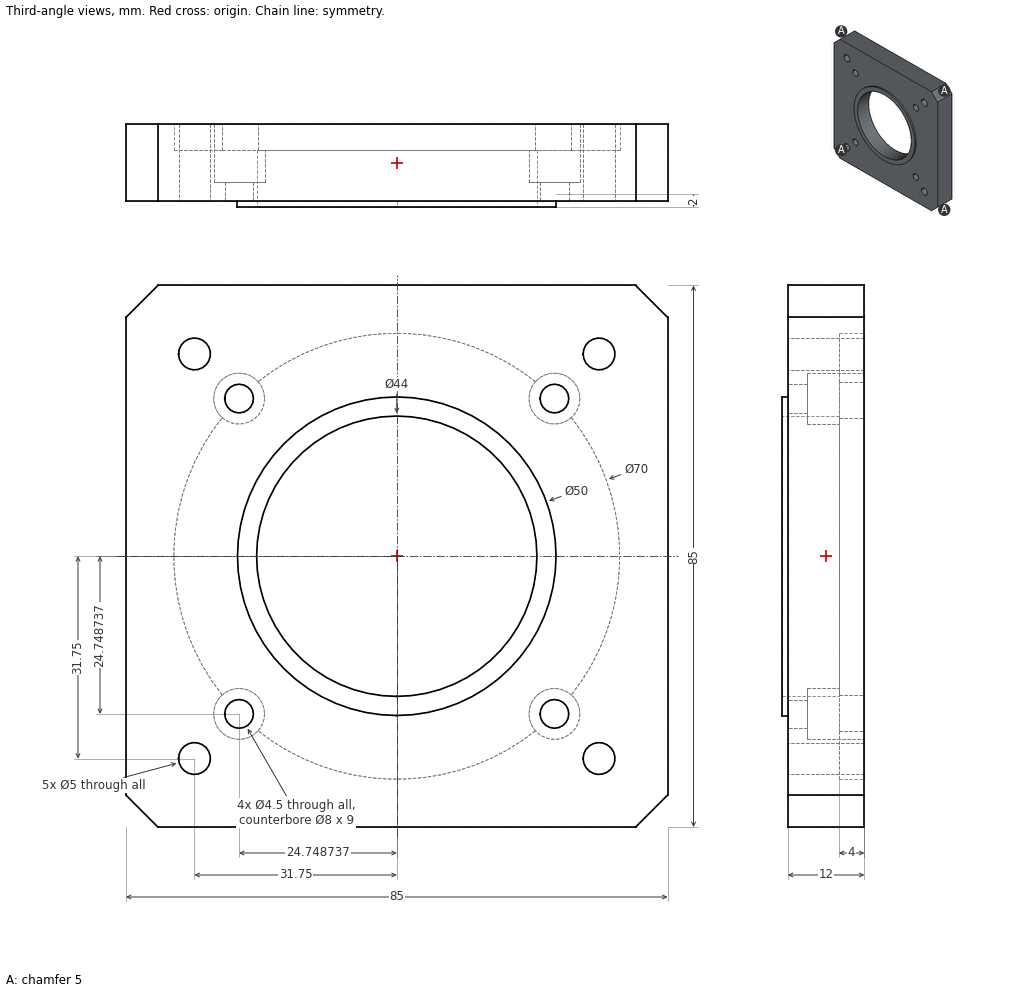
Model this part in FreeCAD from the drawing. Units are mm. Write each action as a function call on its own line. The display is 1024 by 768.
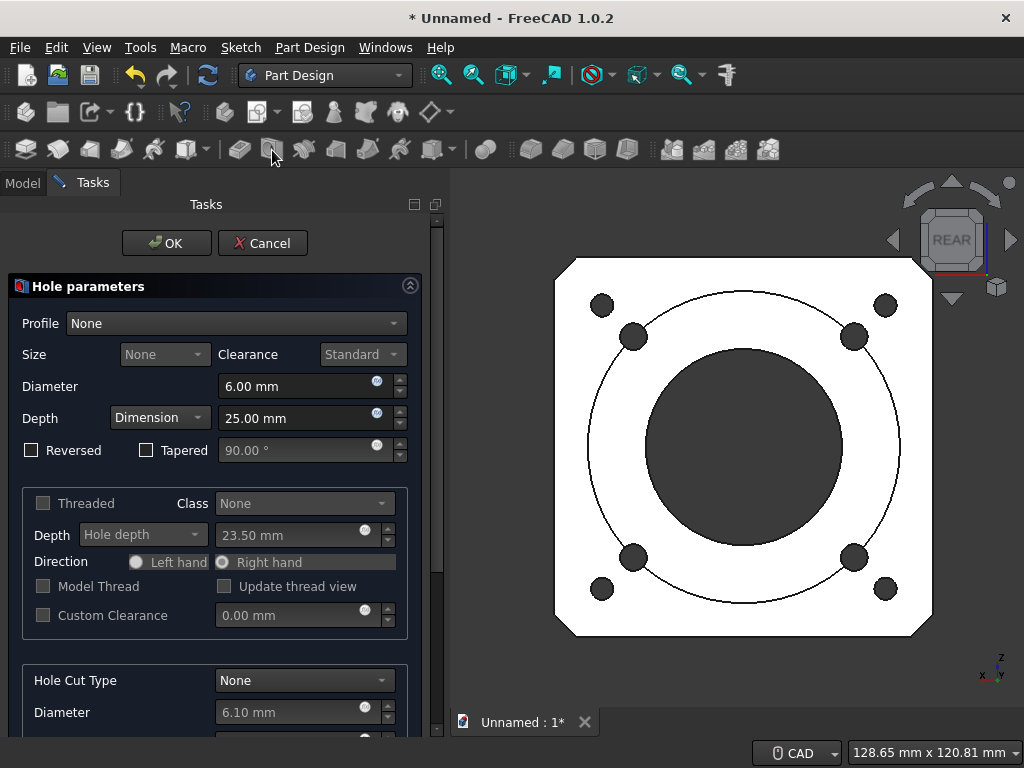
triple_click(305, 386)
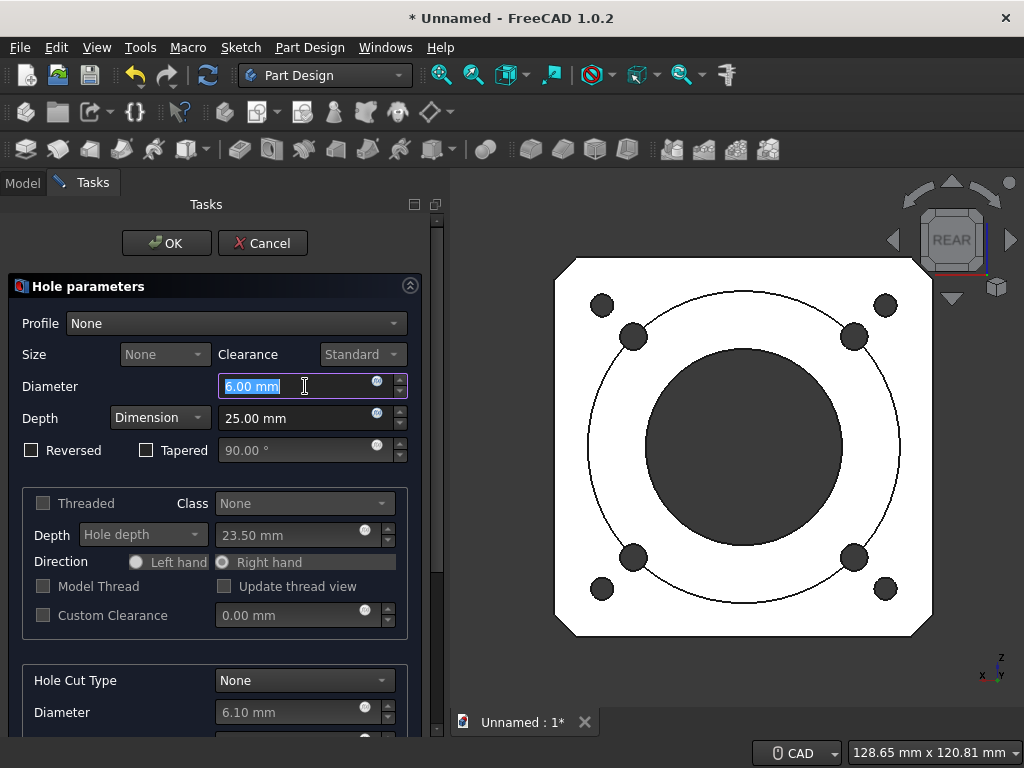
text(4.5)
key(Tab)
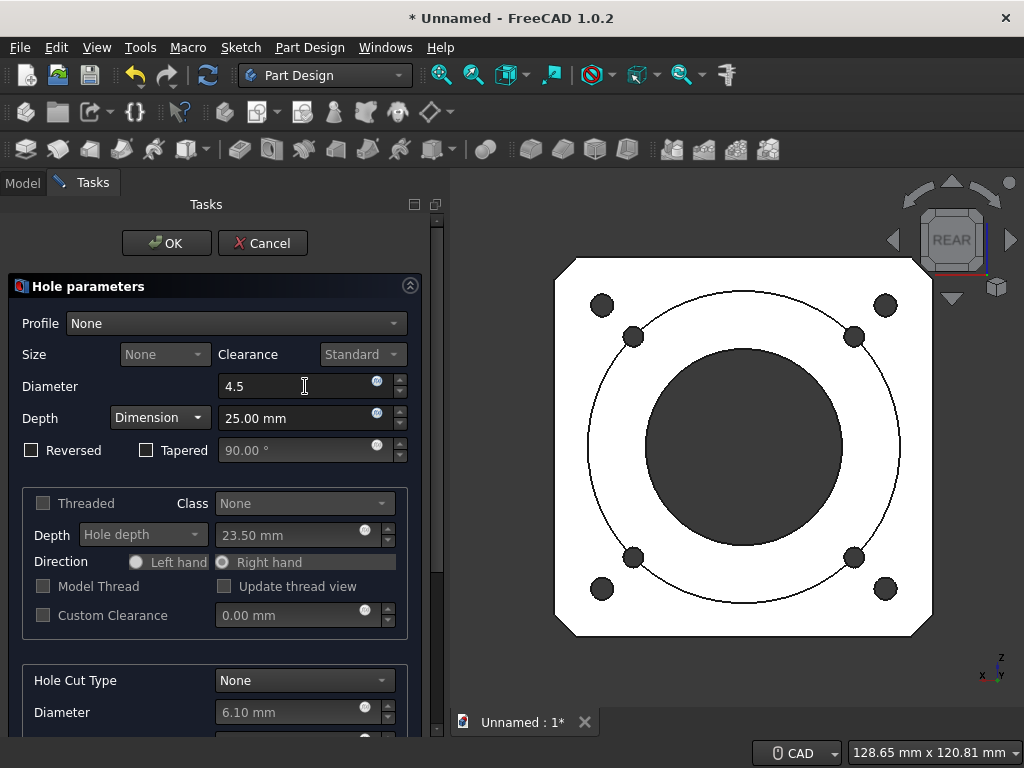
click(161, 418)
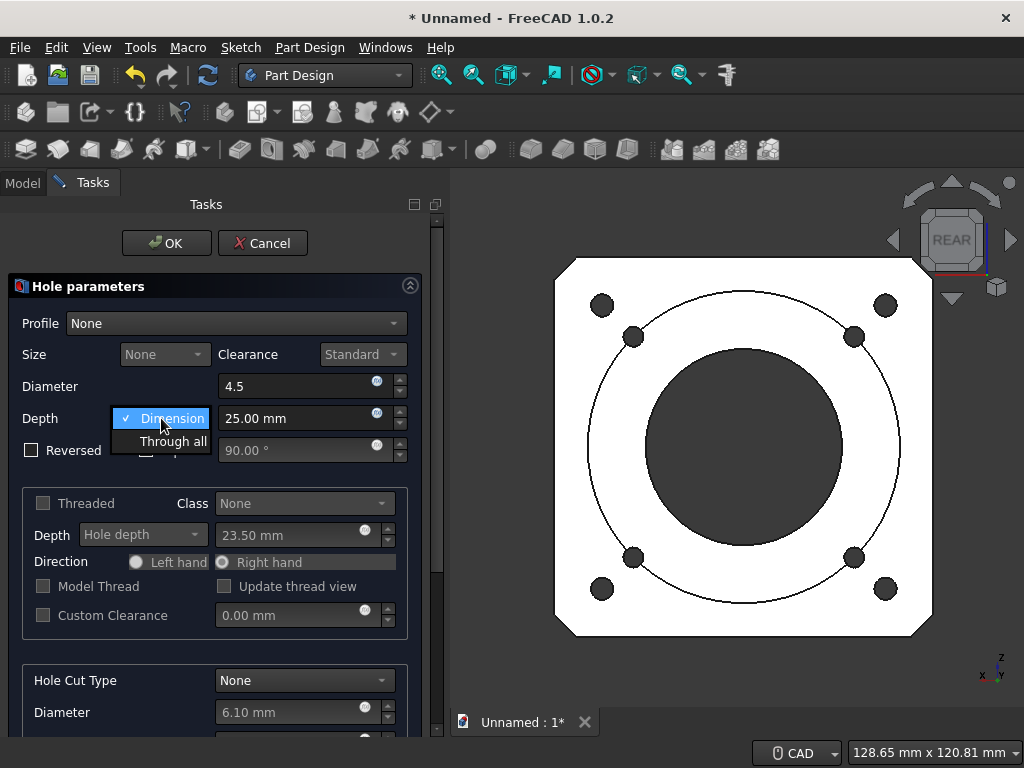
click(160, 442)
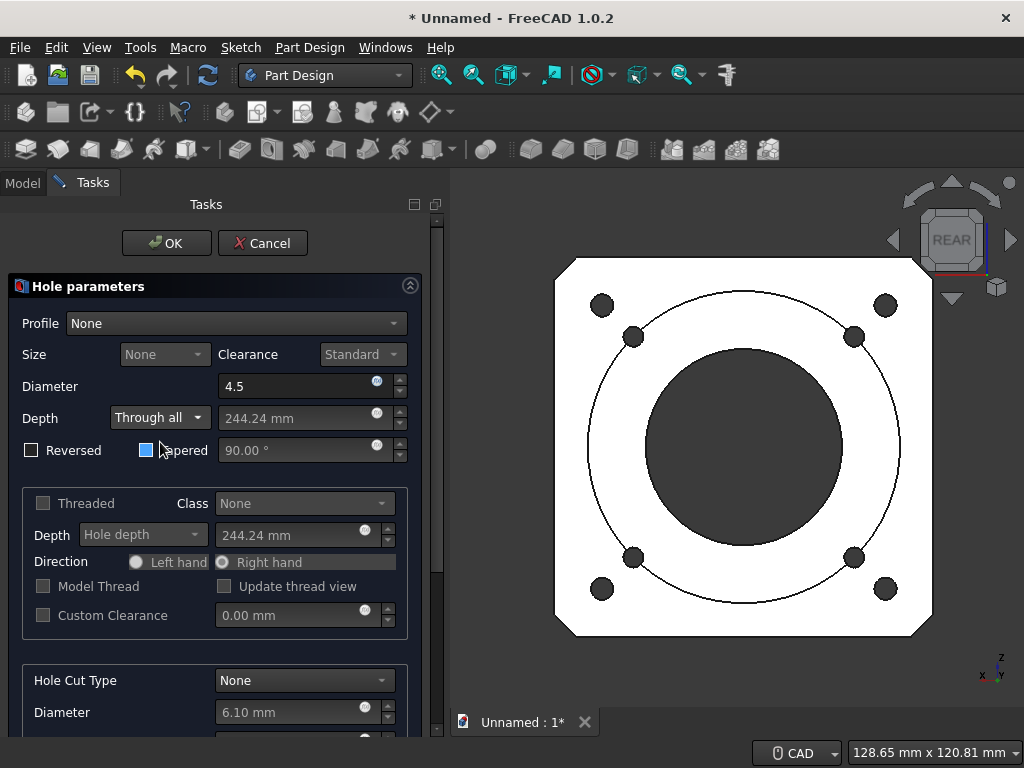
click(306, 680)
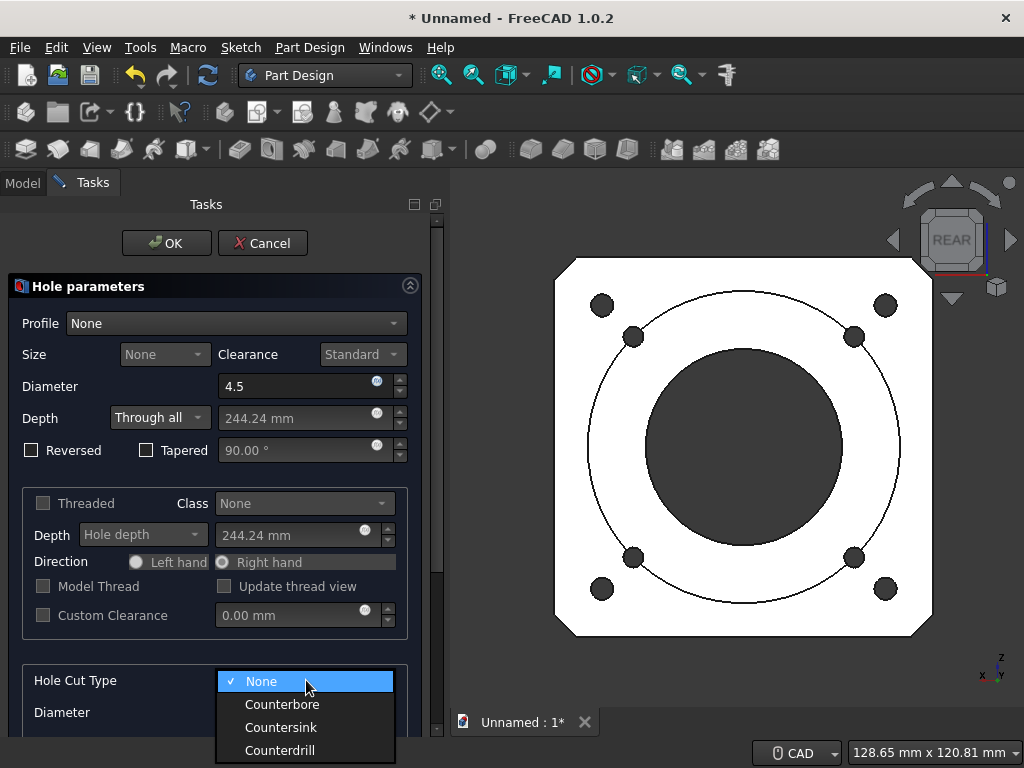
click(304, 704)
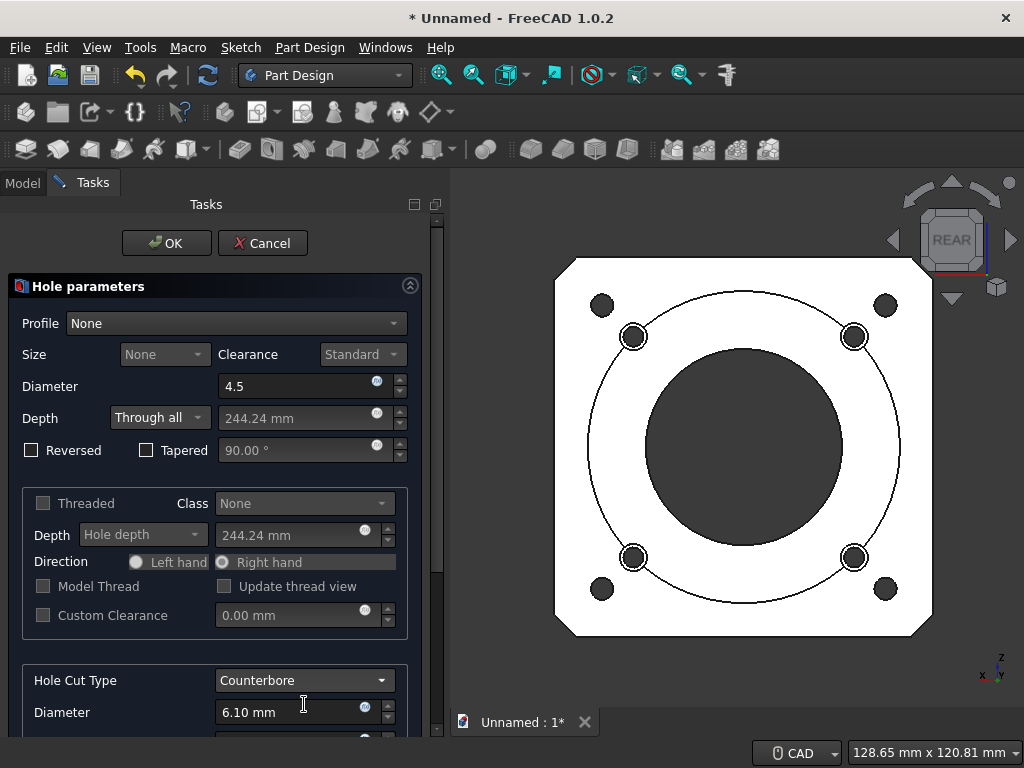
triple_click(298, 712)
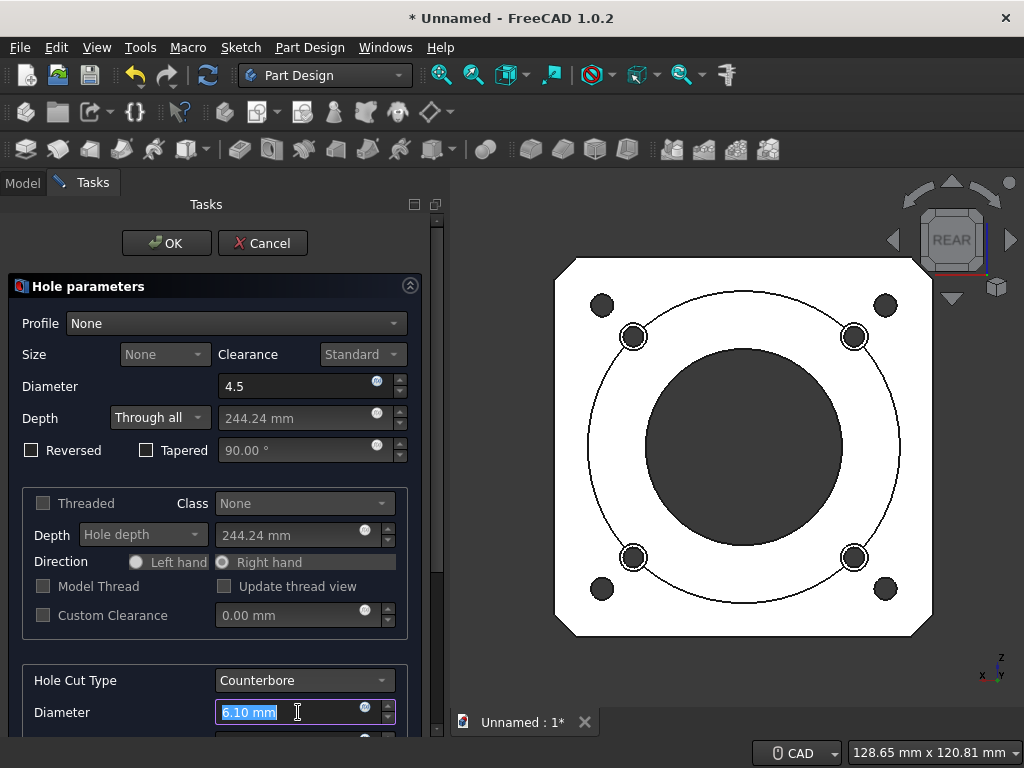
text(8)
key(Tab)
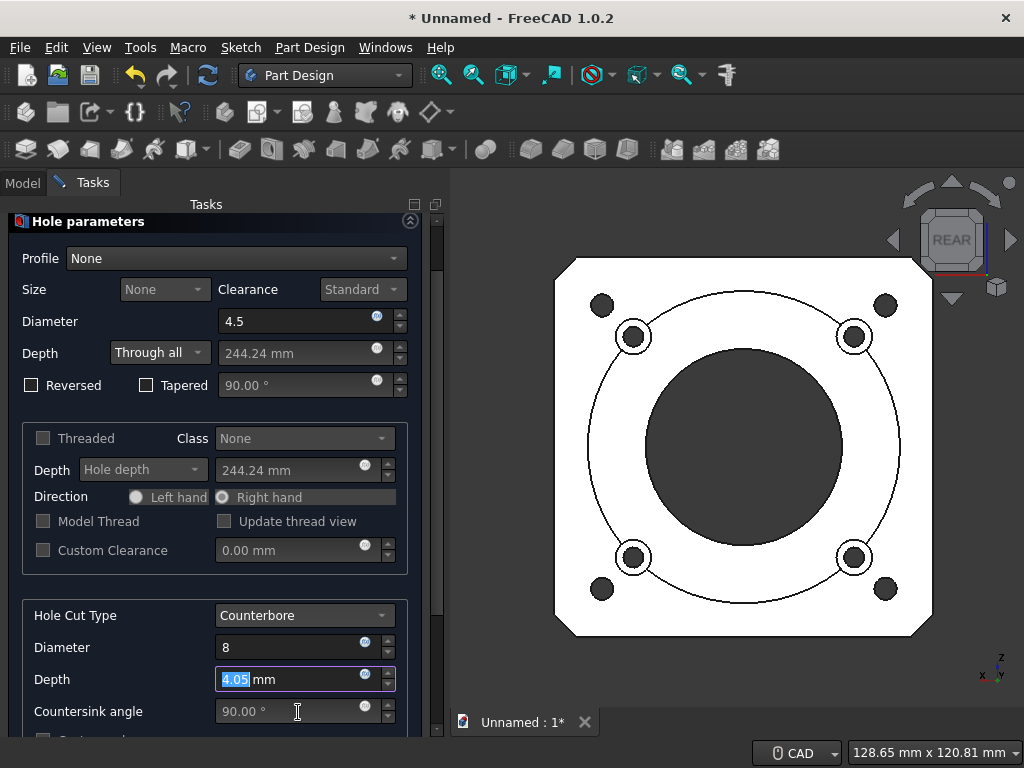
text(9)
key(Tab)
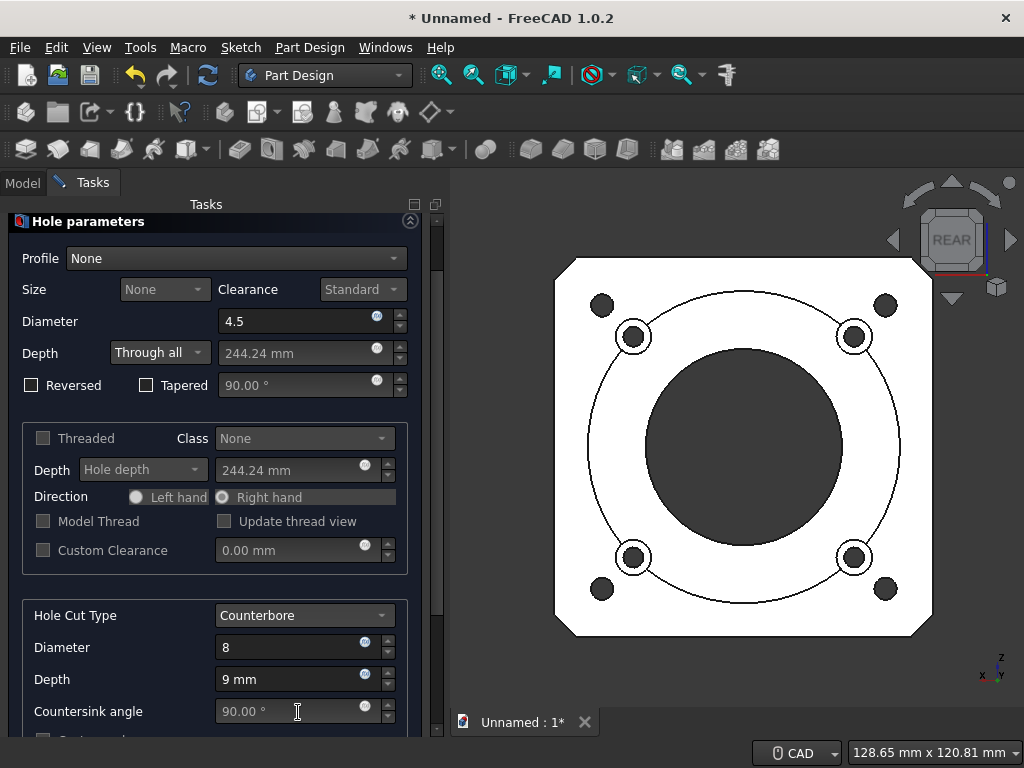
scroll(437, 475, up, 2)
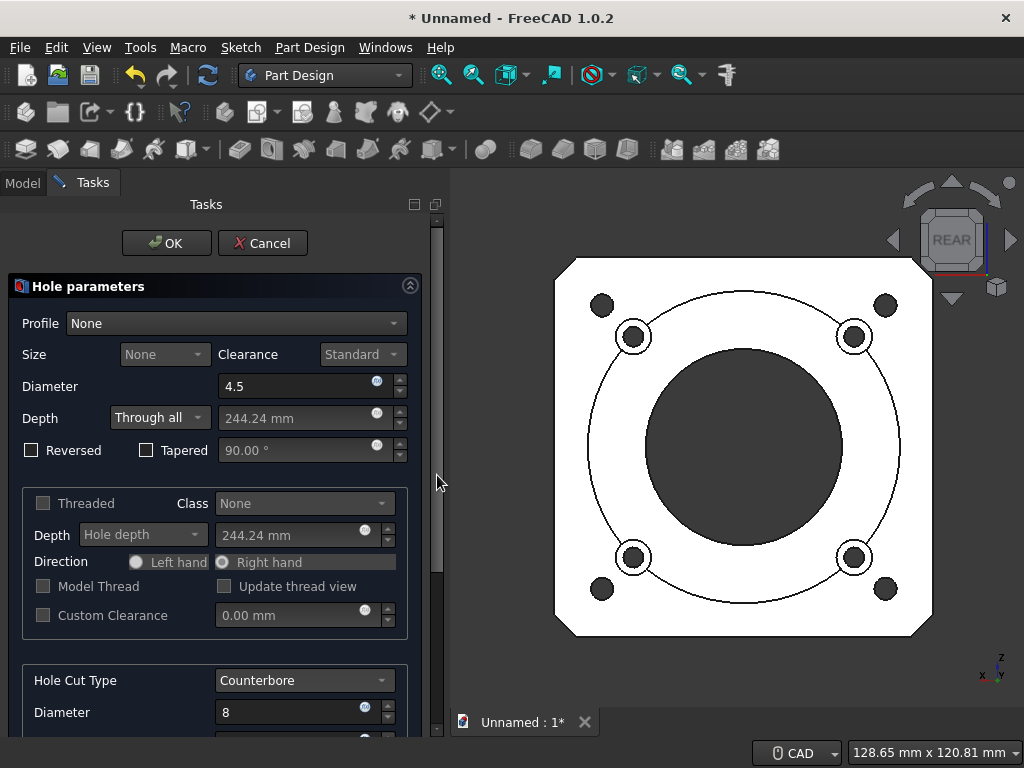
click(167, 243)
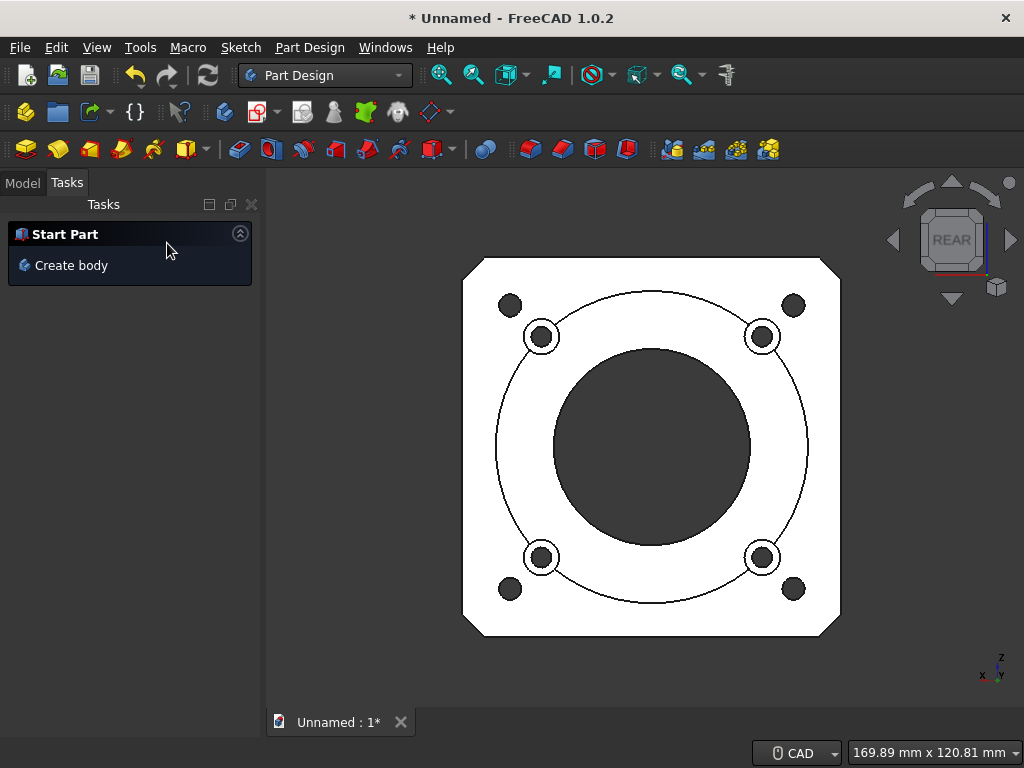
key(0)